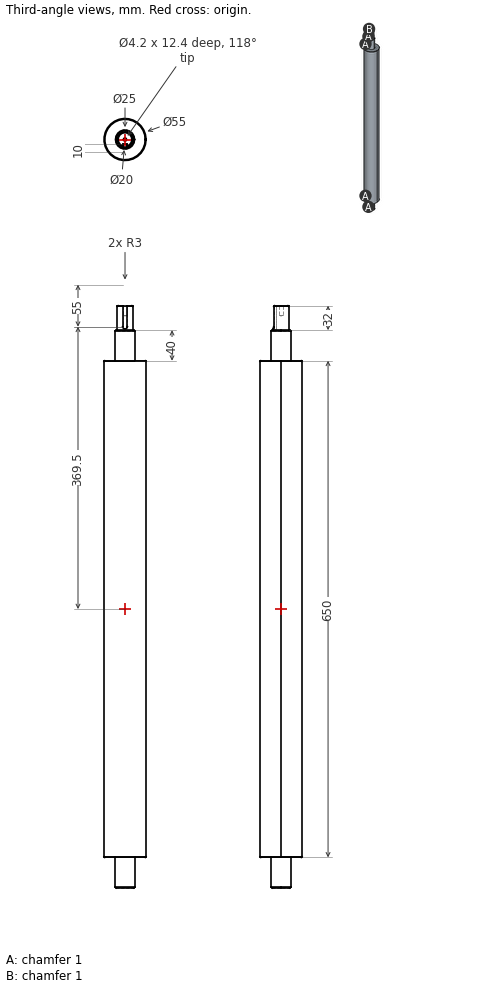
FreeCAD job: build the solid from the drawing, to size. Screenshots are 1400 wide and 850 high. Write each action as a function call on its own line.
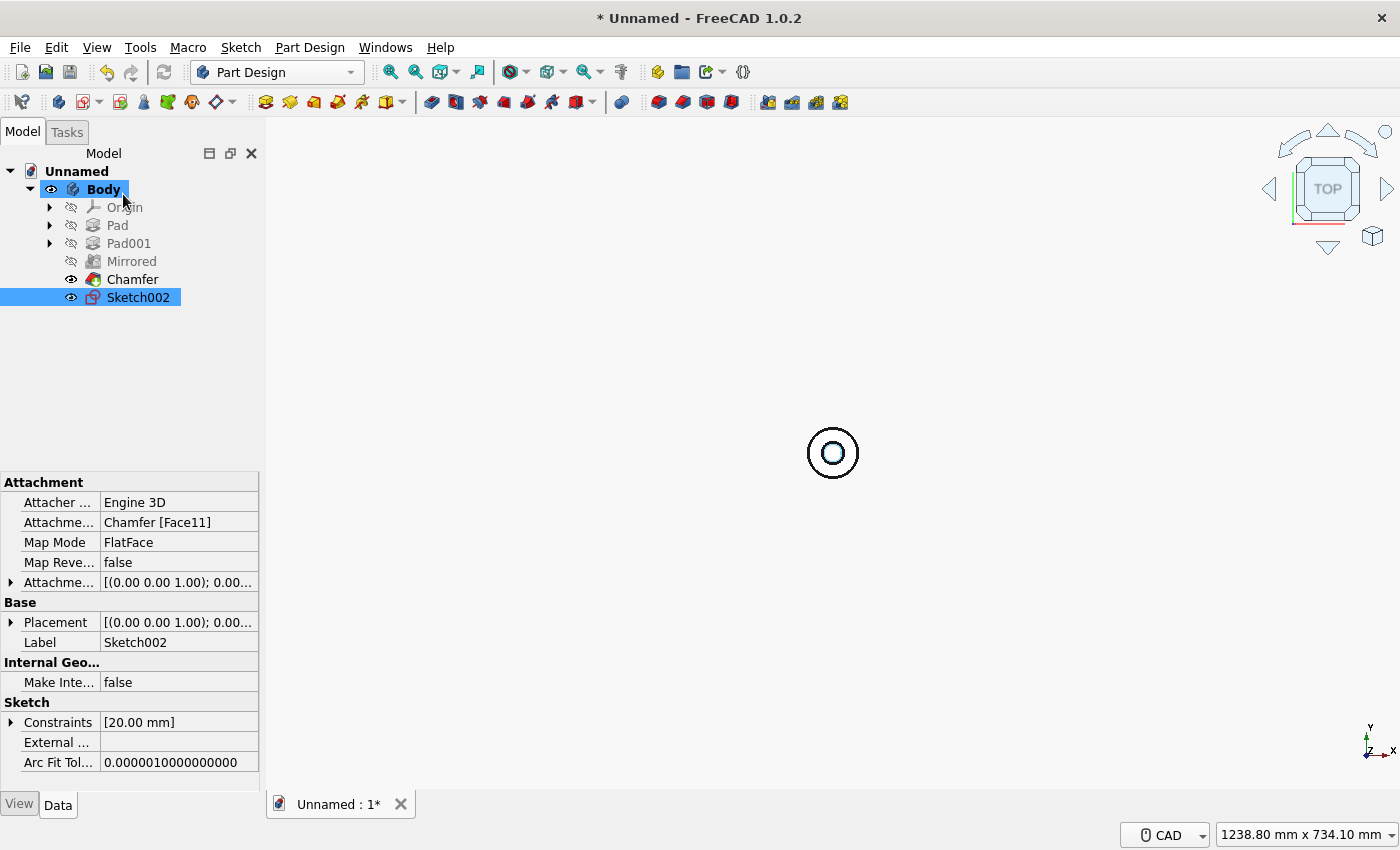
click(266, 102)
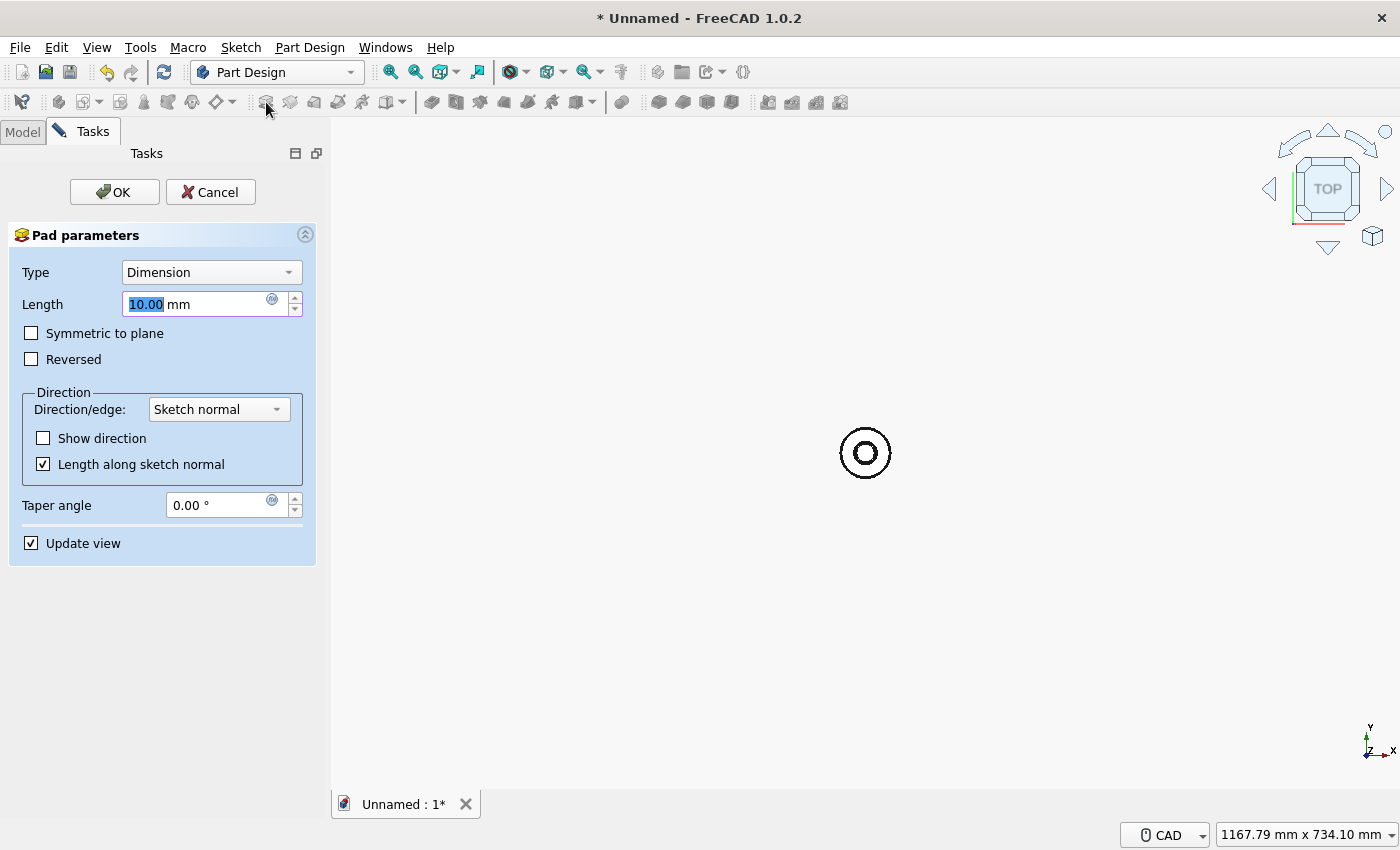
text(32)
key(Tab)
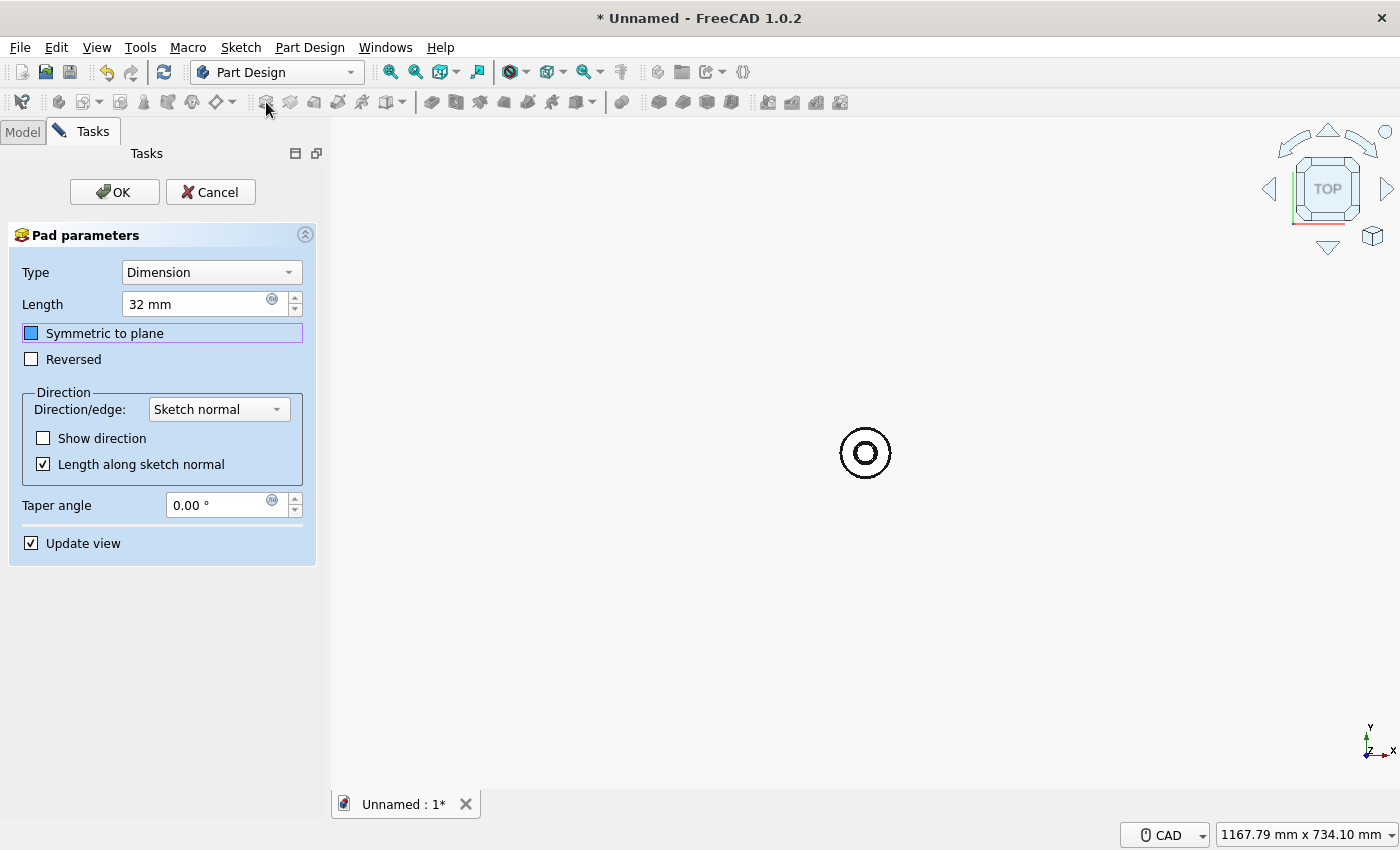
click(115, 192)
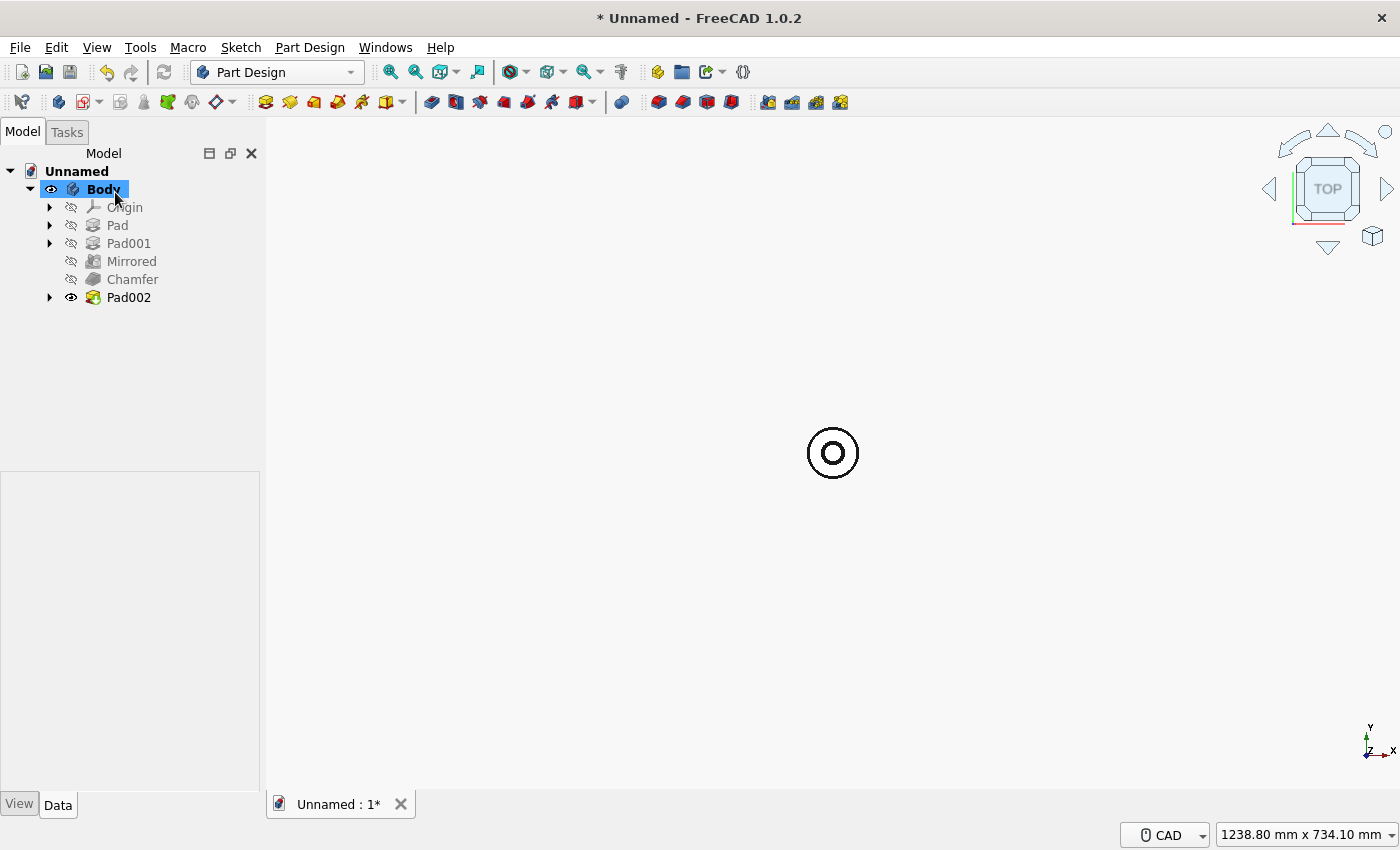
click(392, 72)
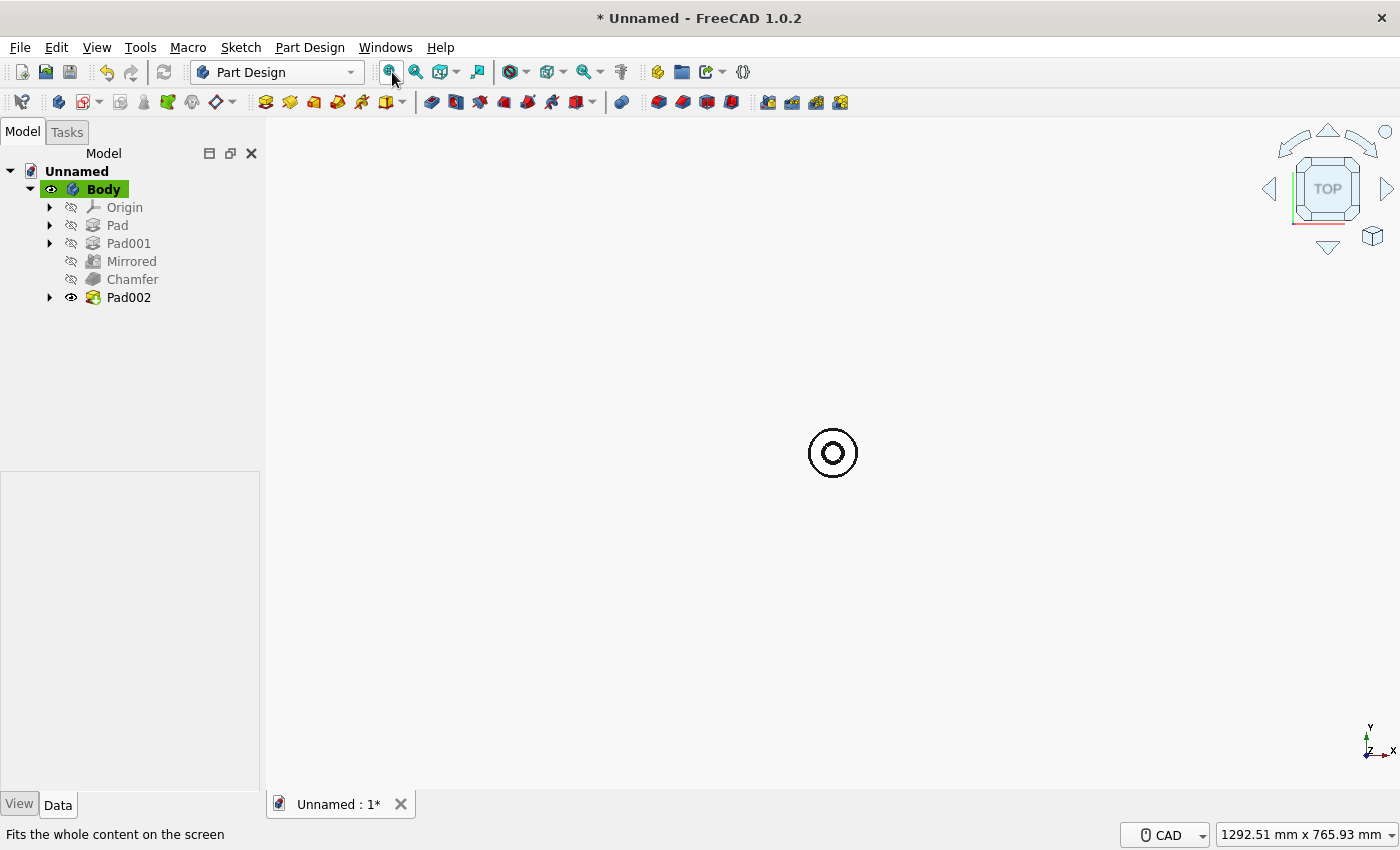
click(824, 452)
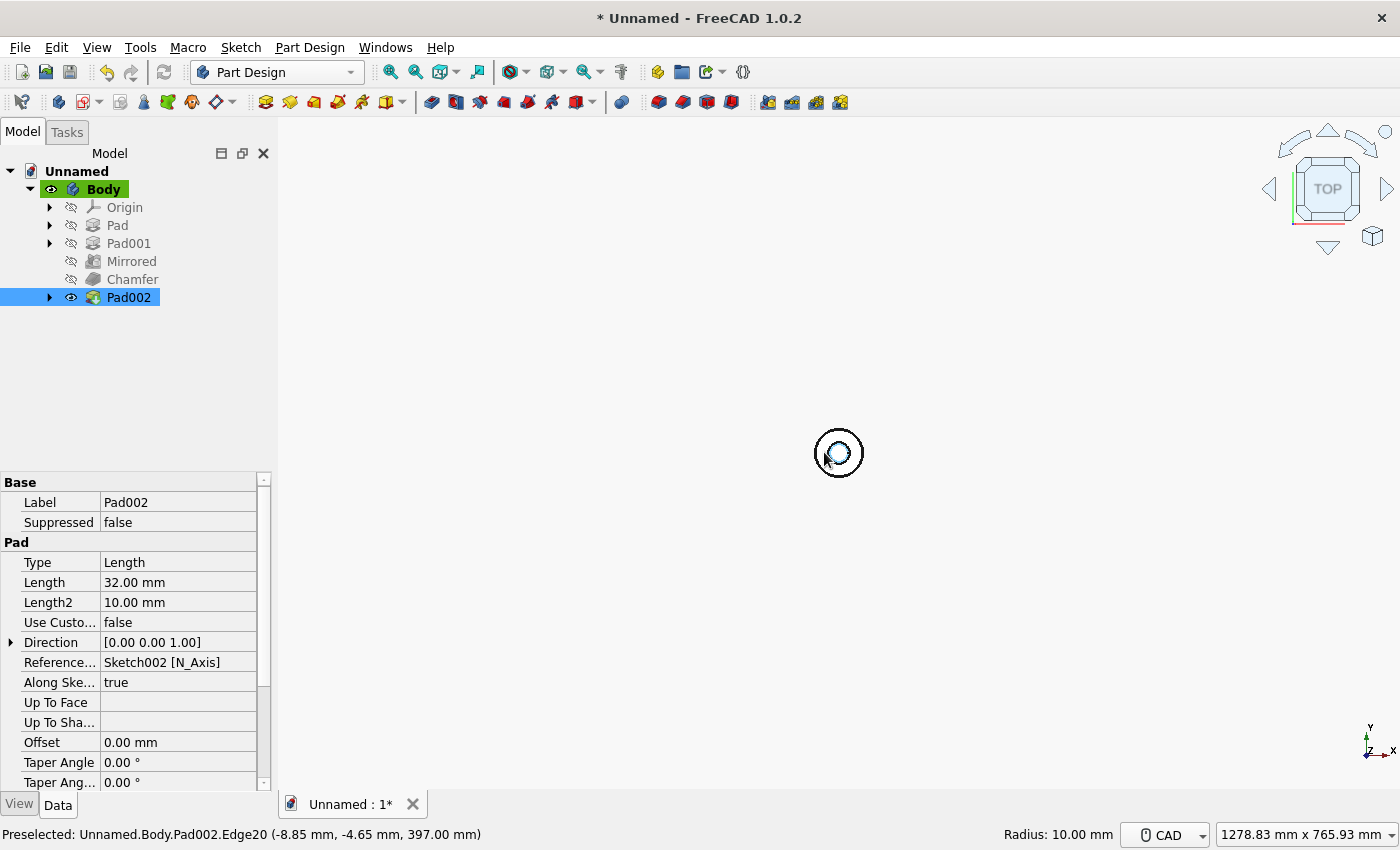
click(684, 102)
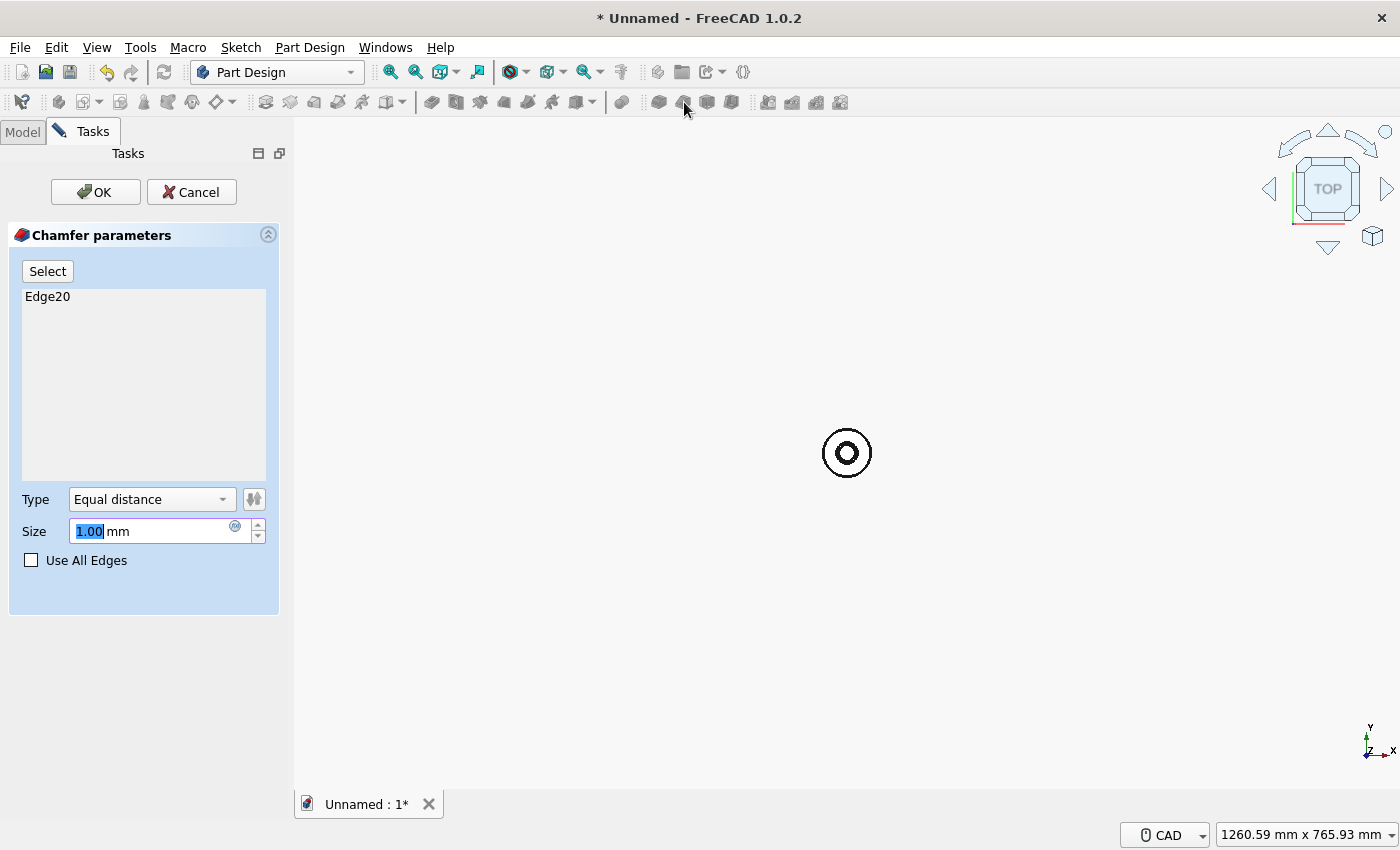
text(1)
key(Tab)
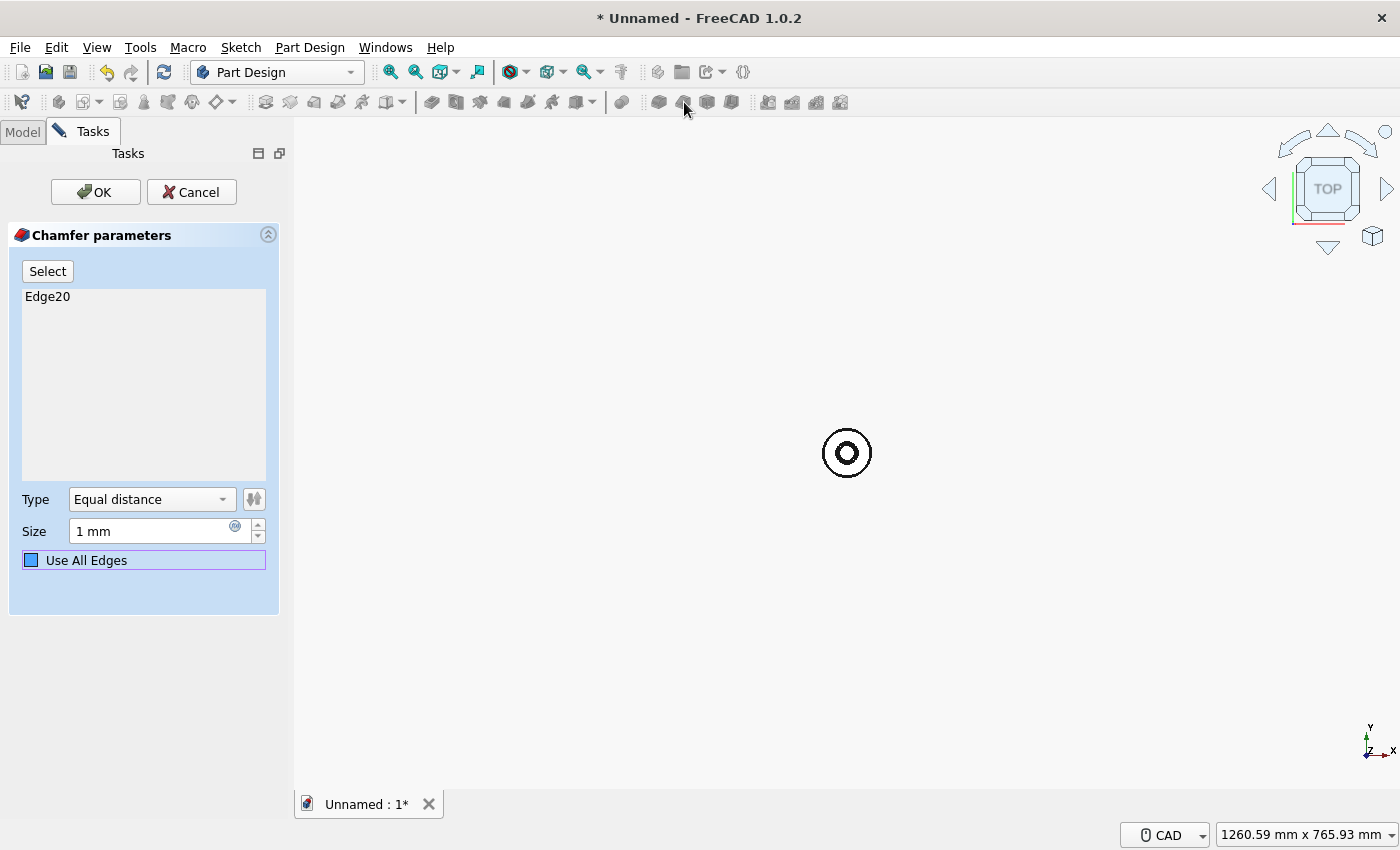
click(96, 192)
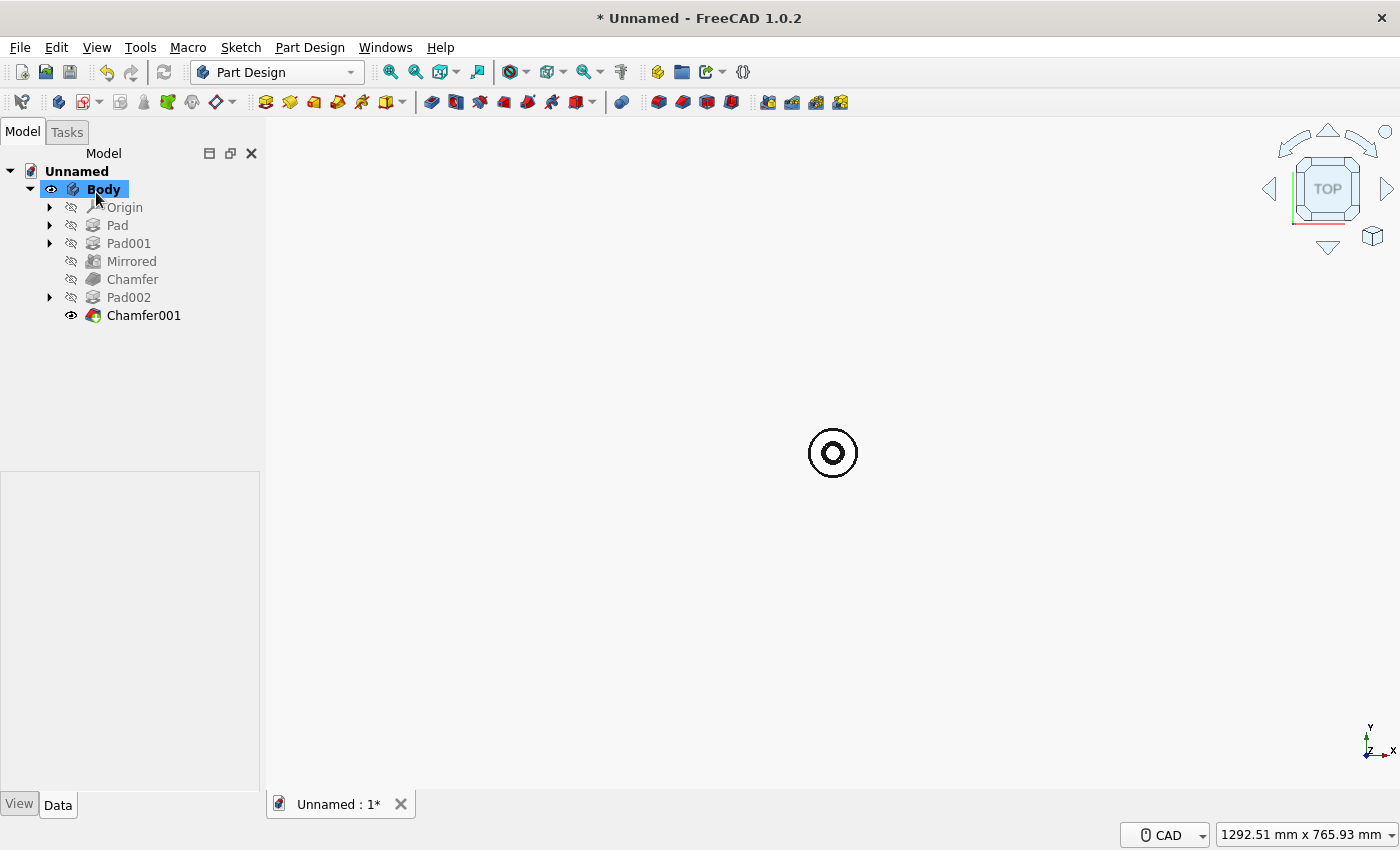
click(392, 72)